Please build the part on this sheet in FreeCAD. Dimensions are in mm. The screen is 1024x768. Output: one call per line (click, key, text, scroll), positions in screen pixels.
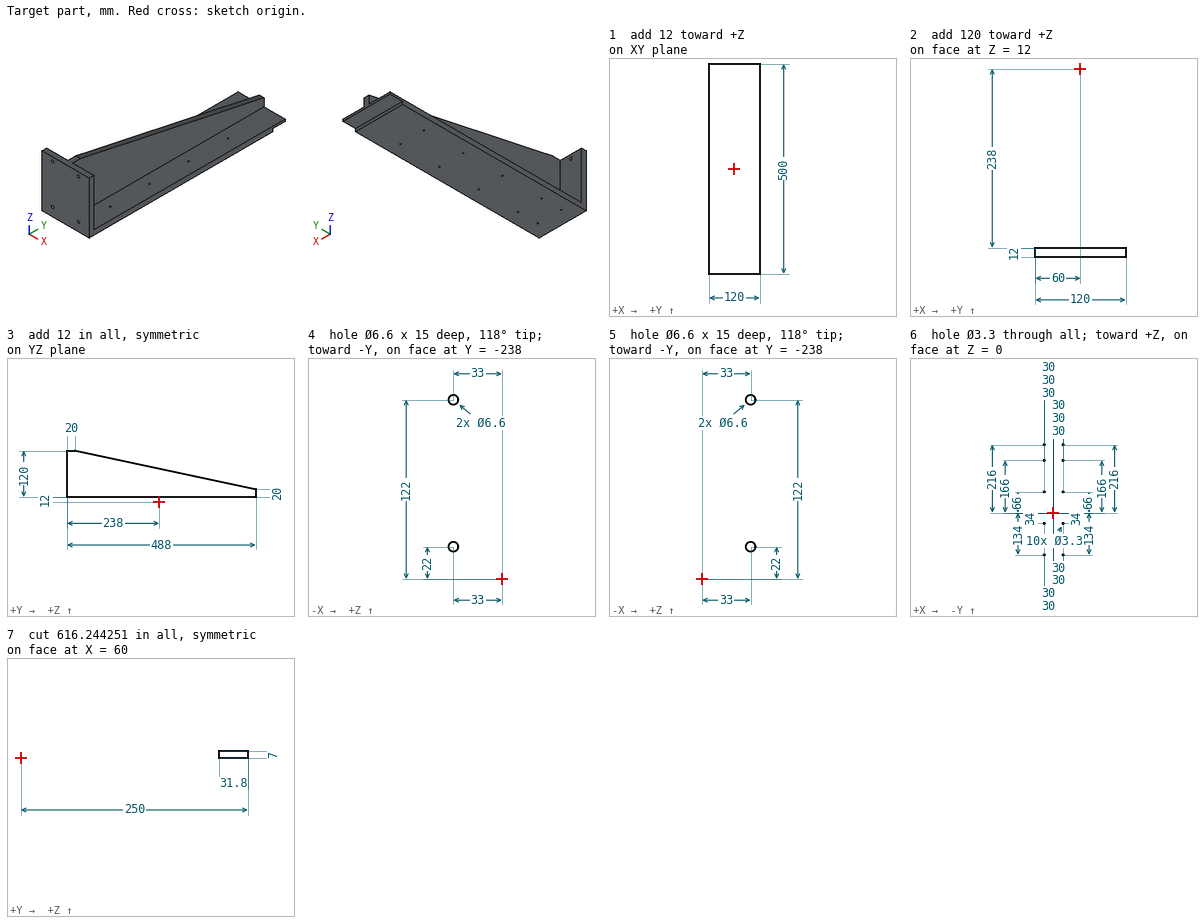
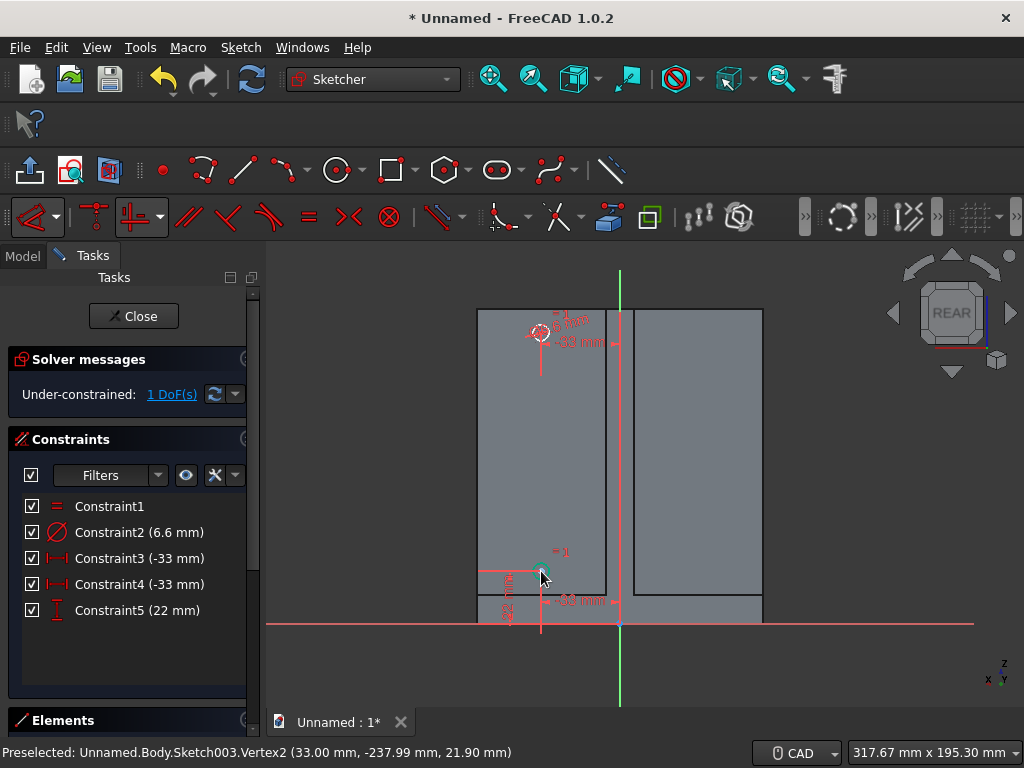
click(541, 333)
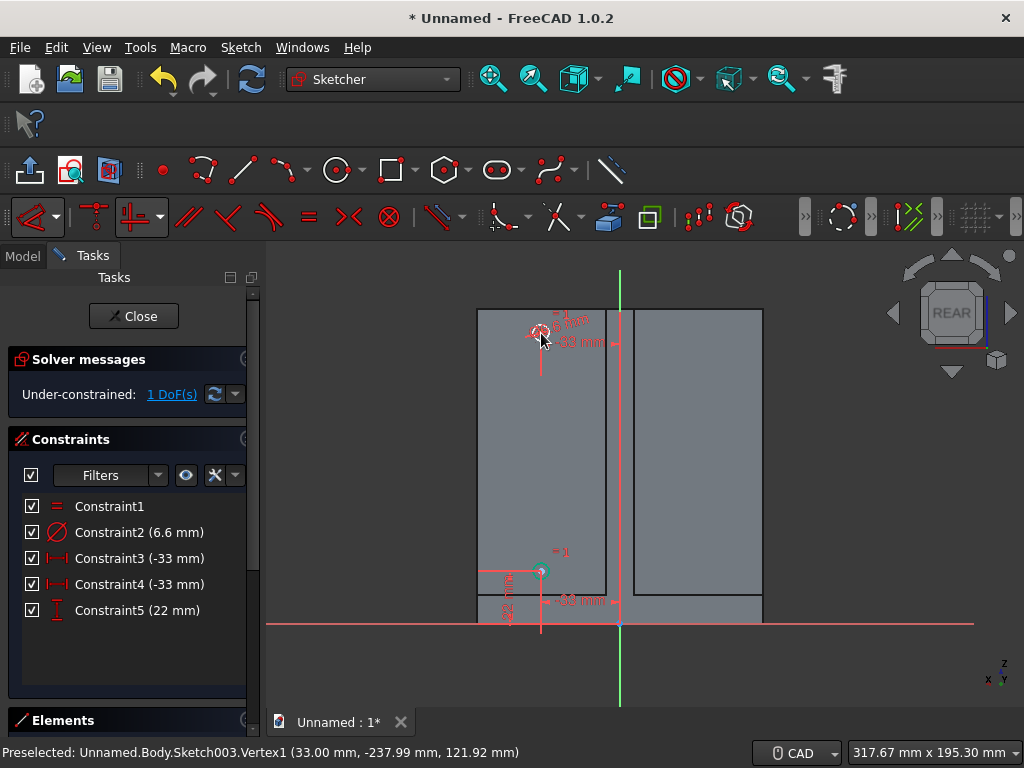
click(58, 218)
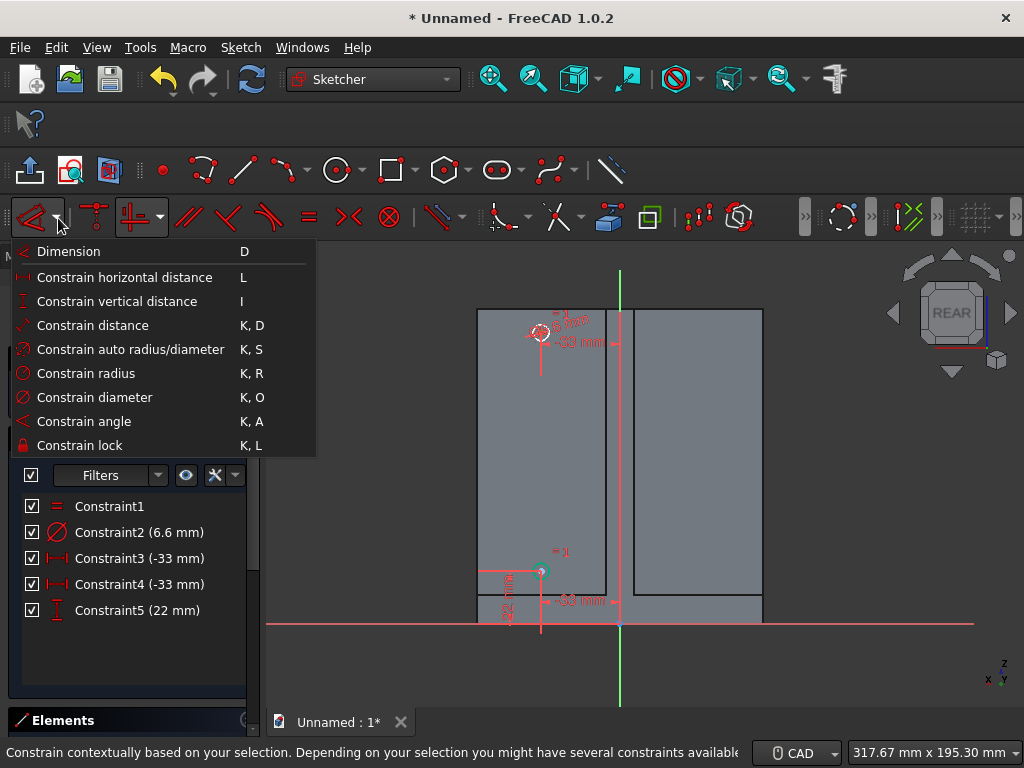
click(164, 301)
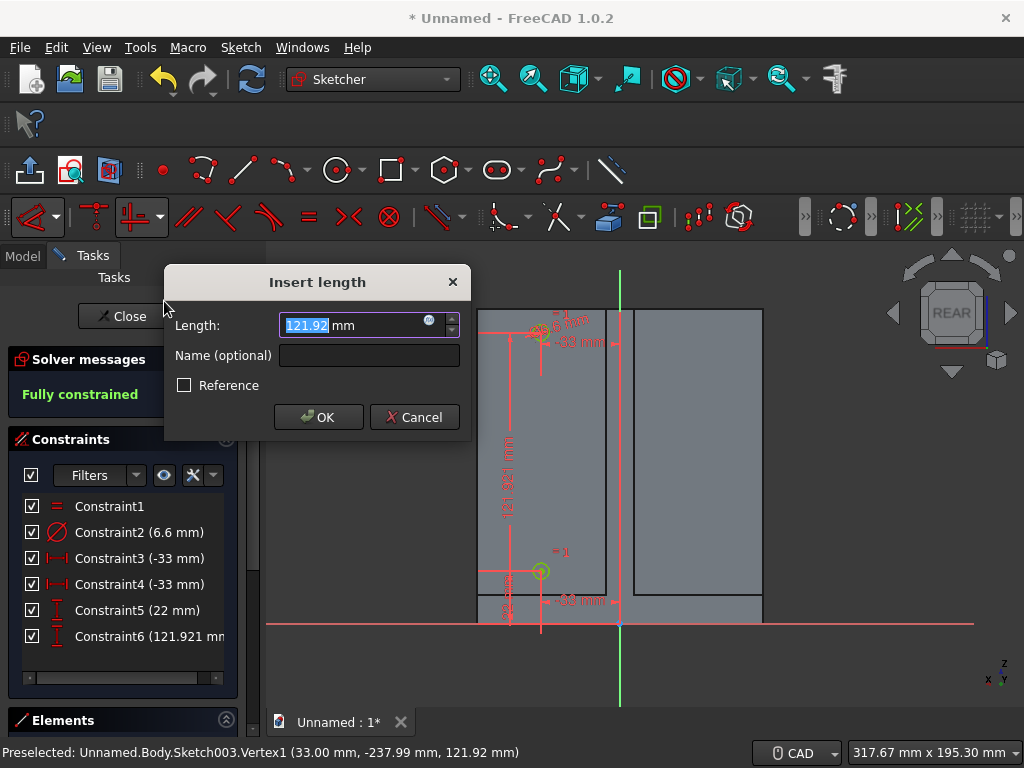
text(122)
key(Return)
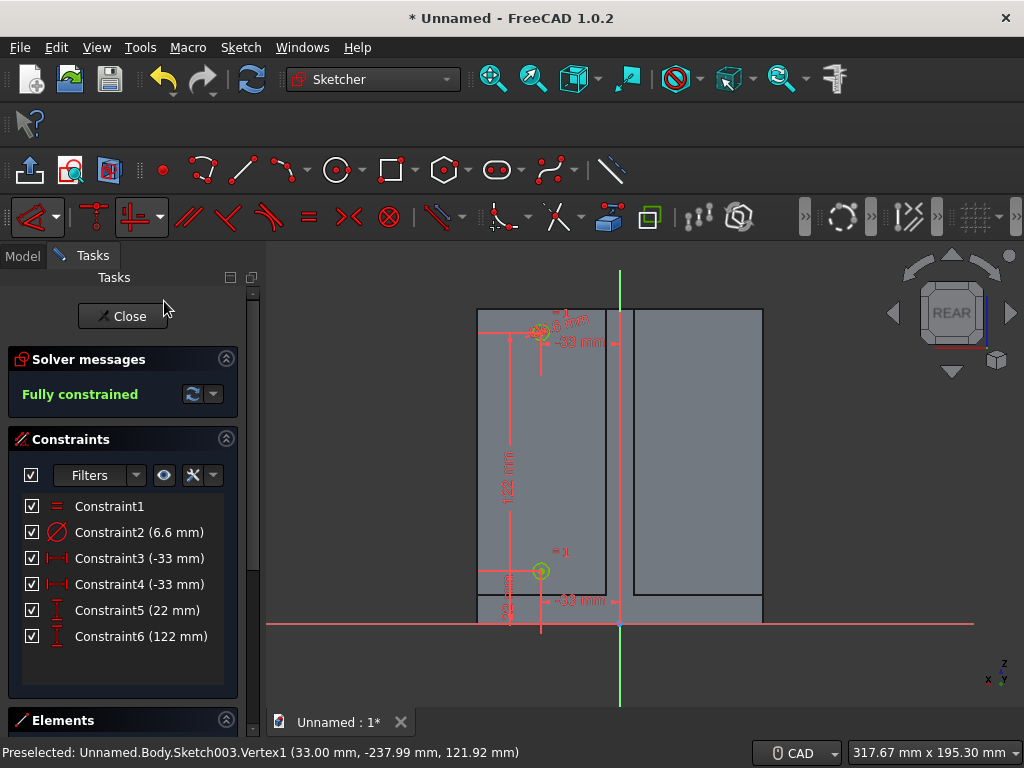
click(123, 316)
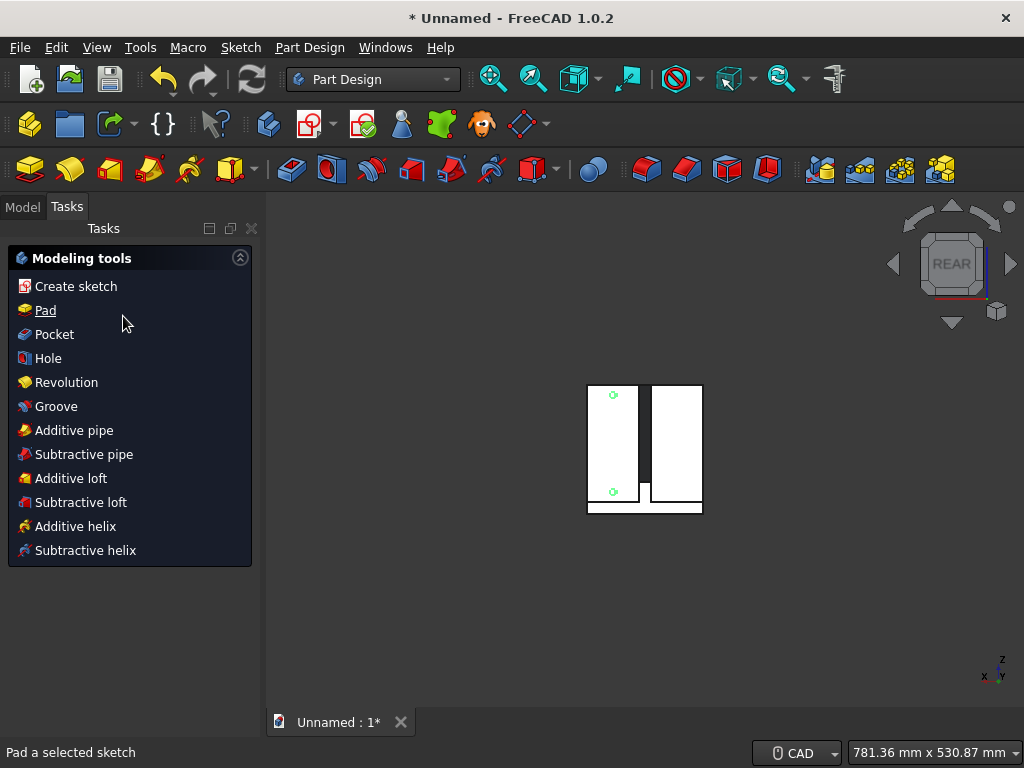
click(332, 170)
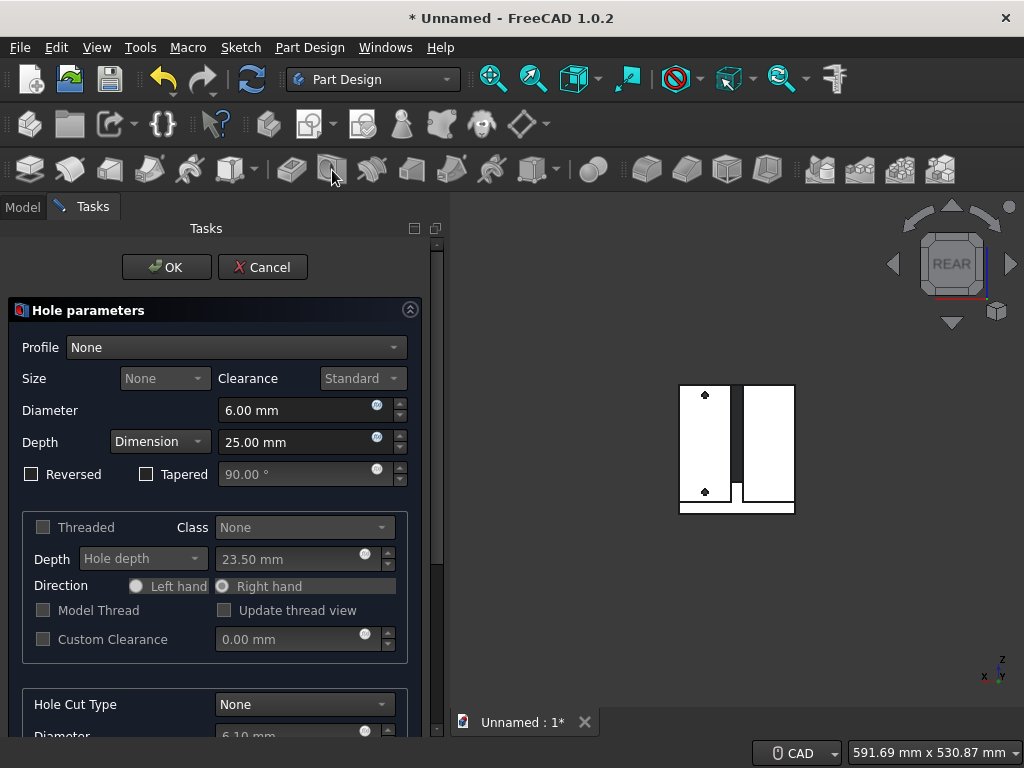
triple_click(305, 410)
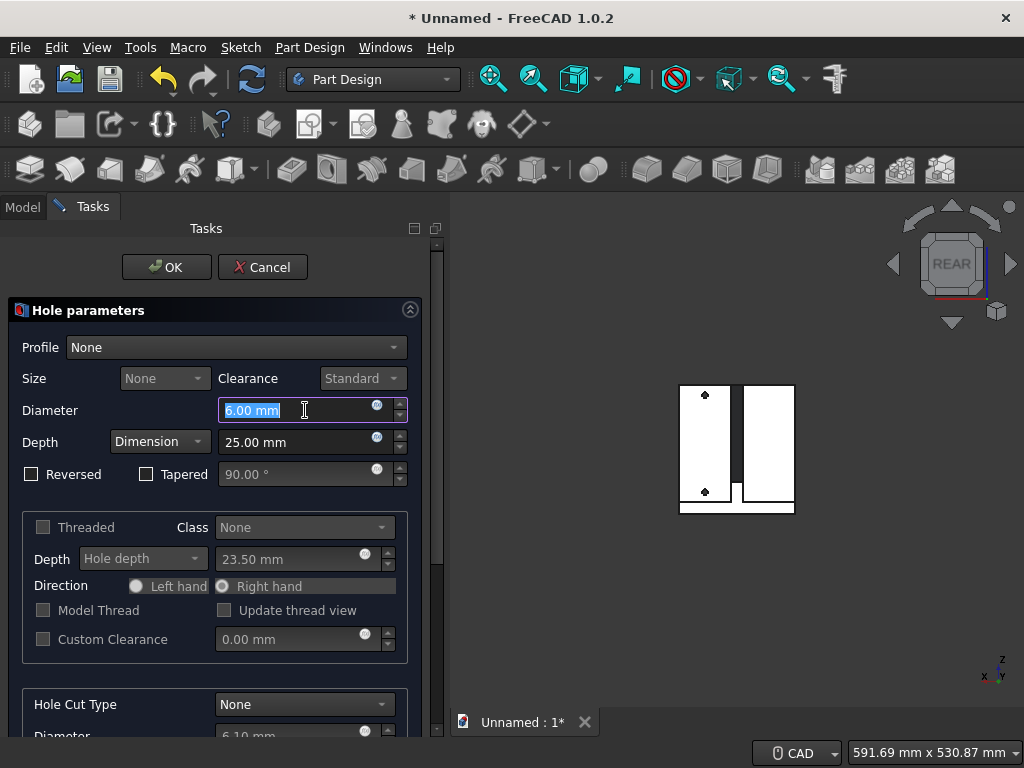
text(6.6)
key(Tab)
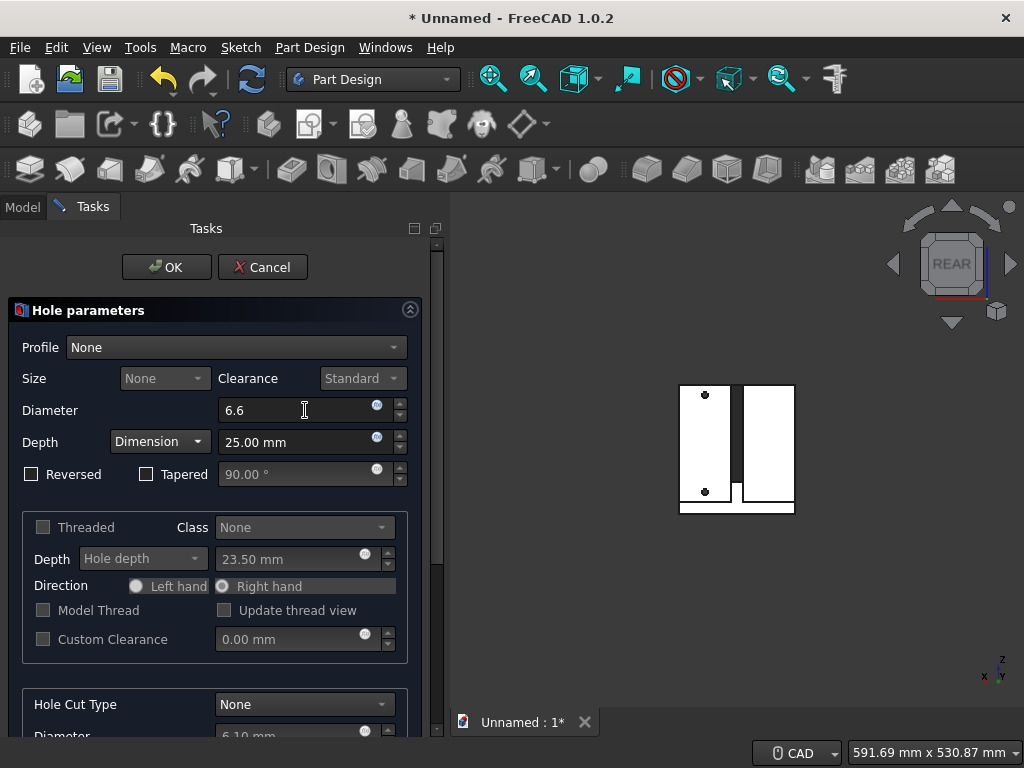
triple_click(305, 442)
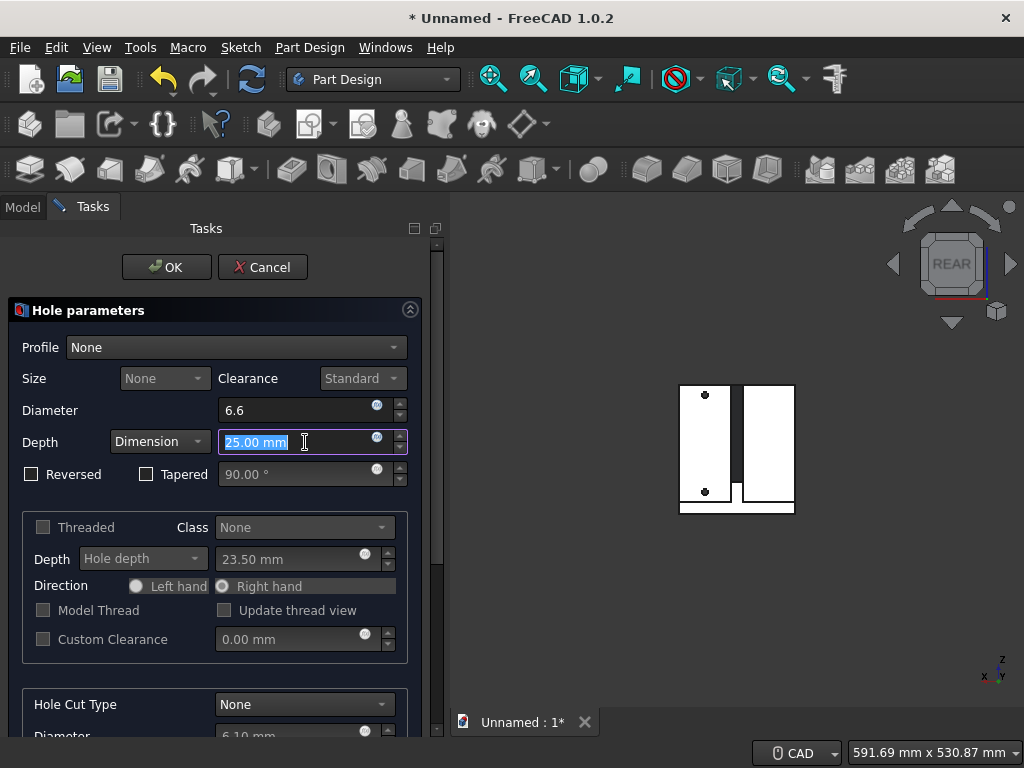
text(15)
key(Tab)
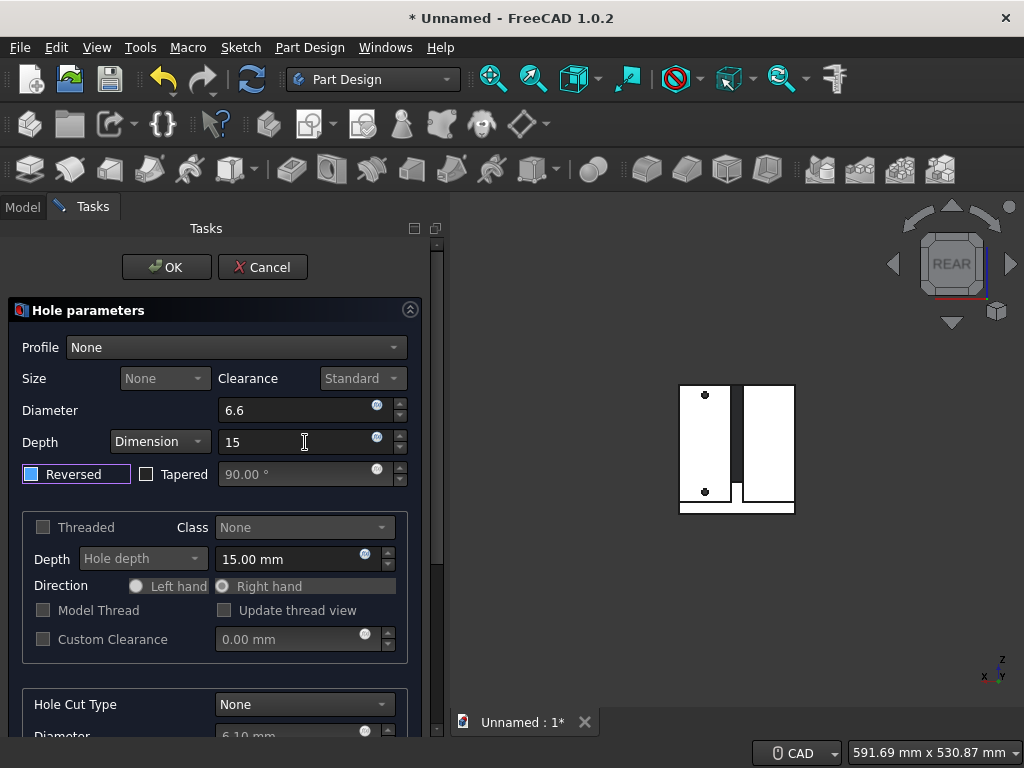
click(167, 267)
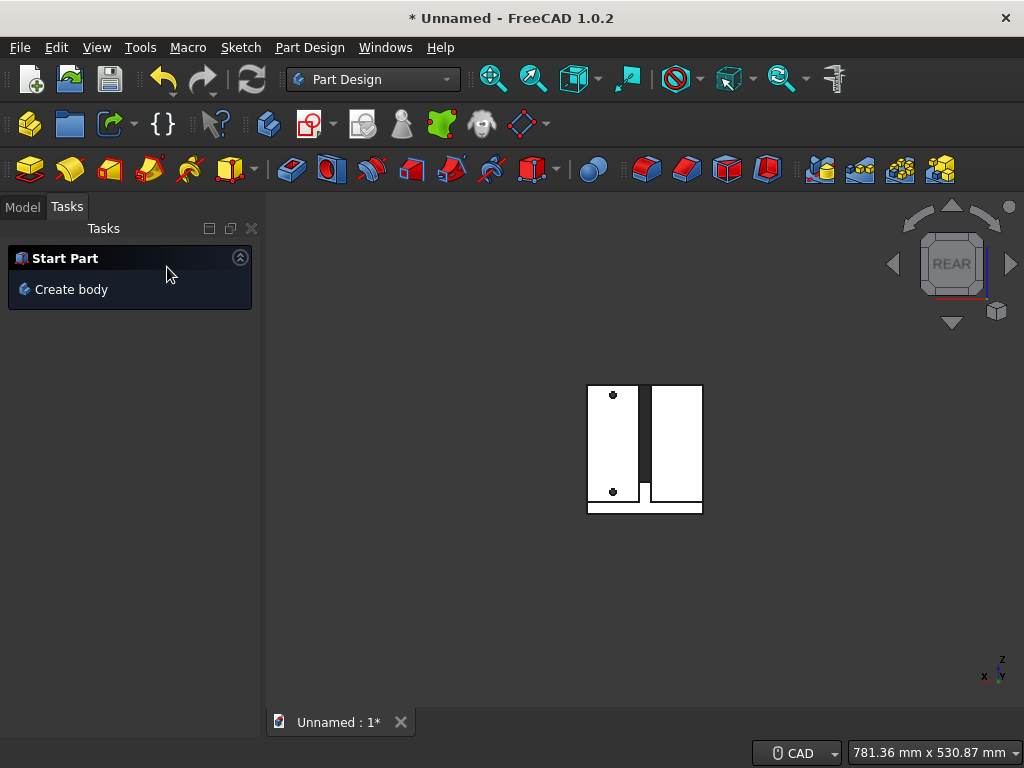
click(494, 80)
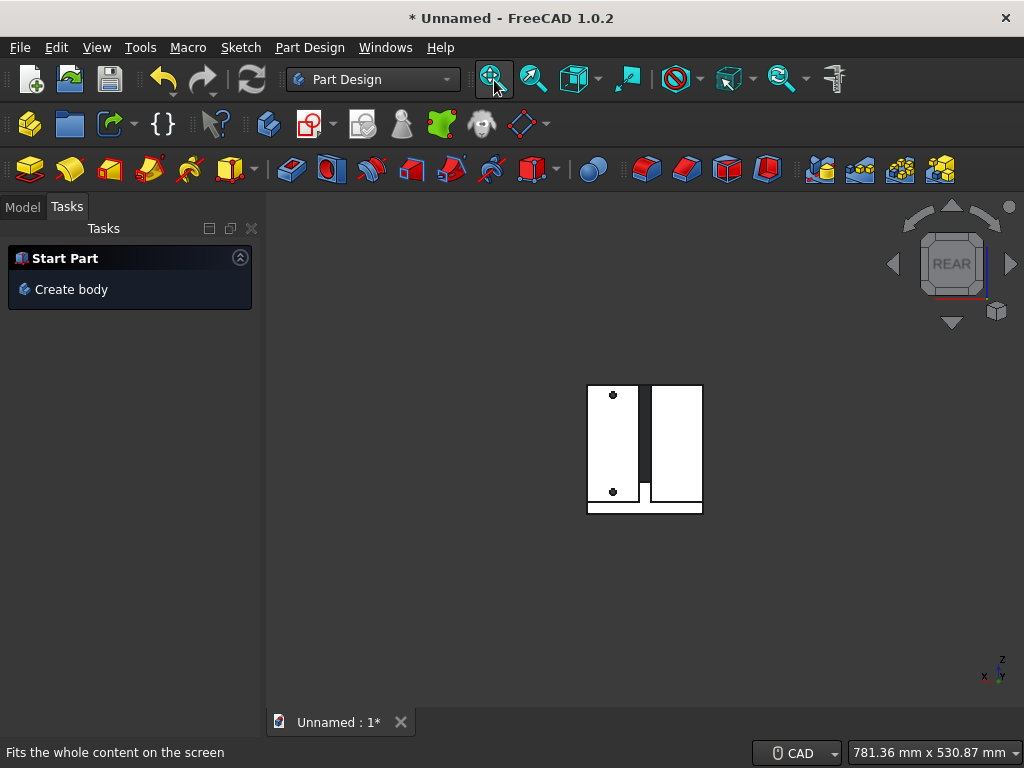
click(677, 426)